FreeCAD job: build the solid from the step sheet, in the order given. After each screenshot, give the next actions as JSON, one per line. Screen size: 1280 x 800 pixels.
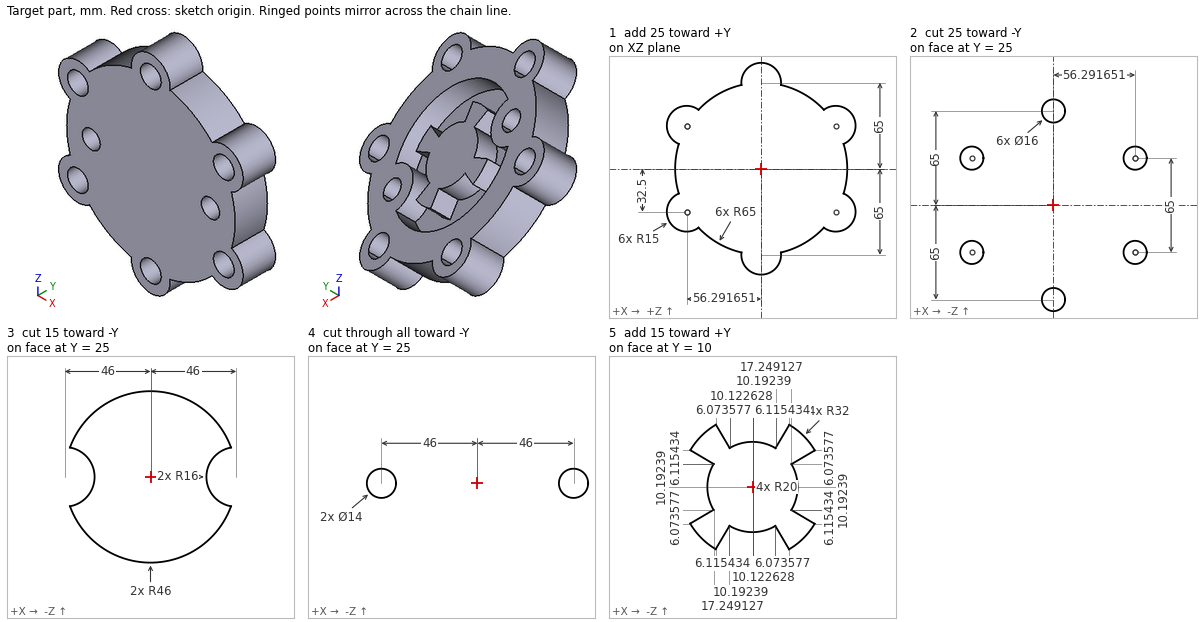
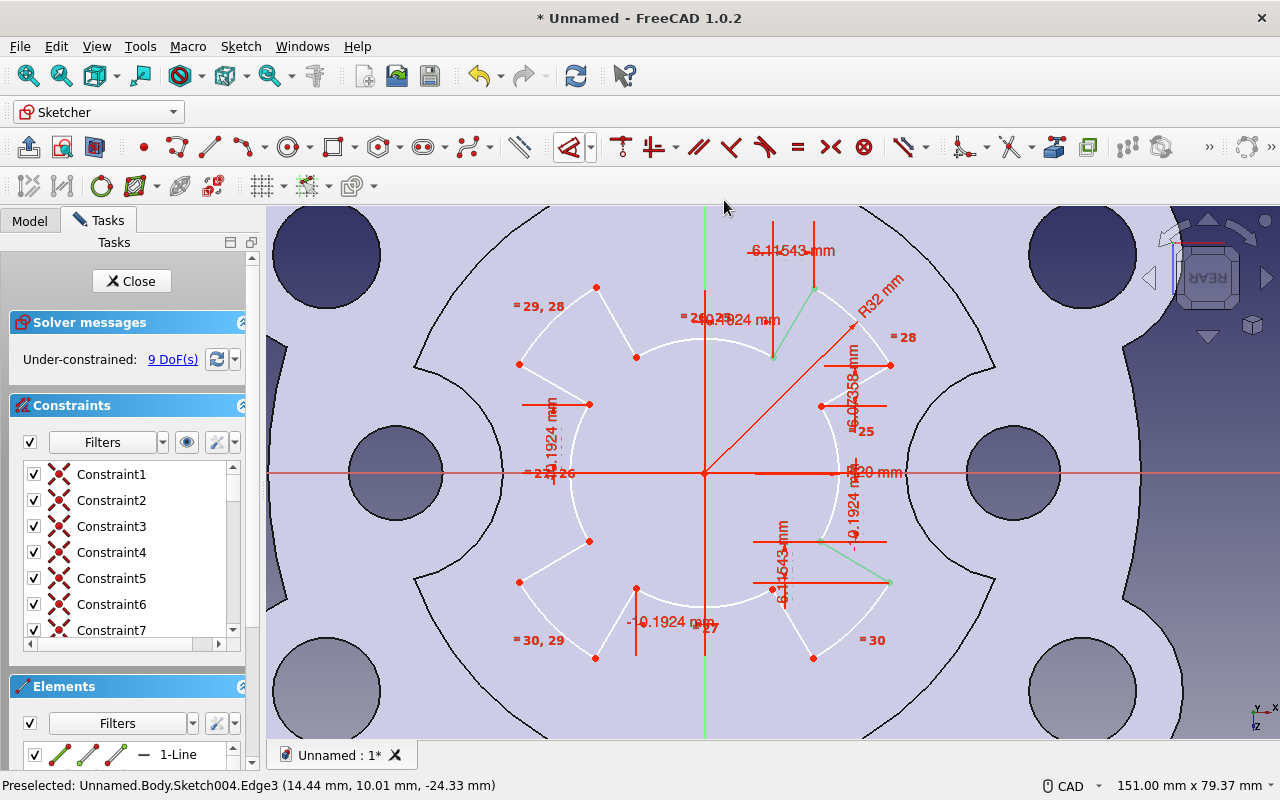
{"action": "left_click", "coordinate": [624, 337]}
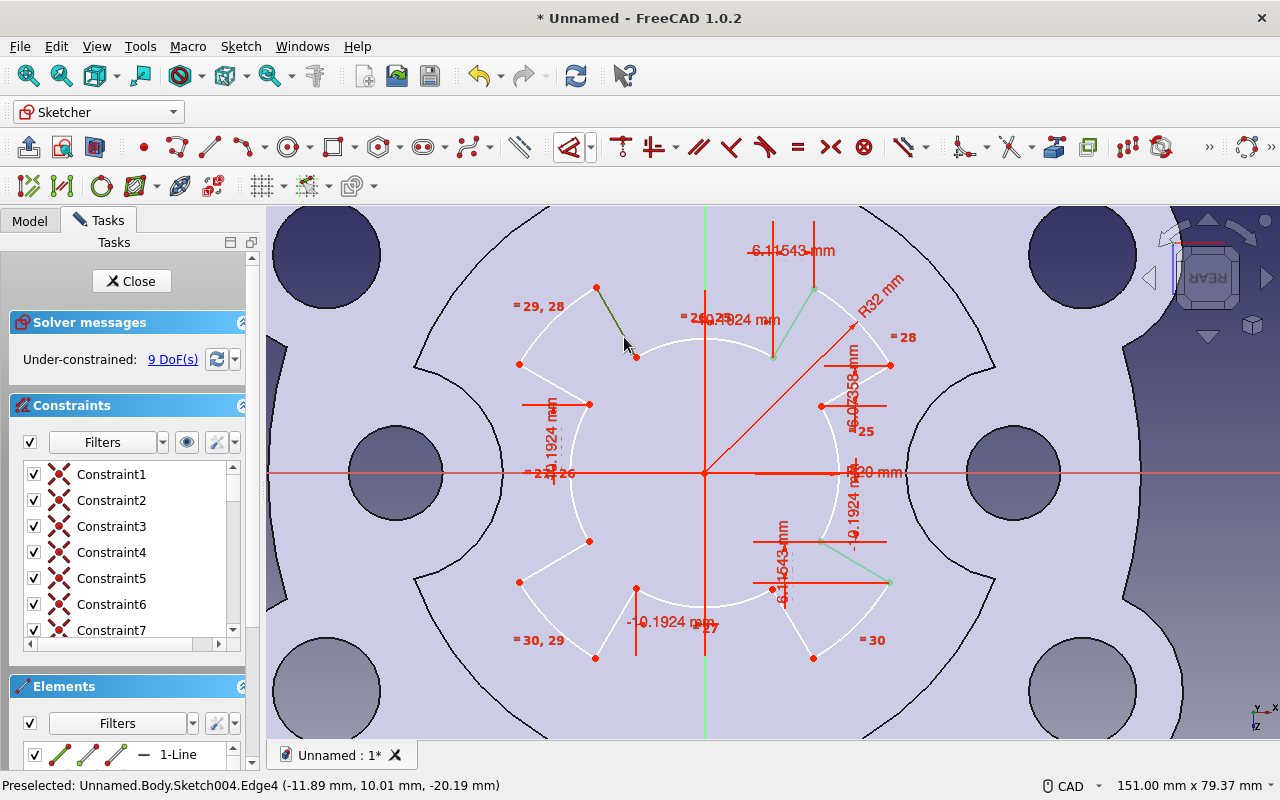
{"action": "left_click", "coordinate": [590, 148]}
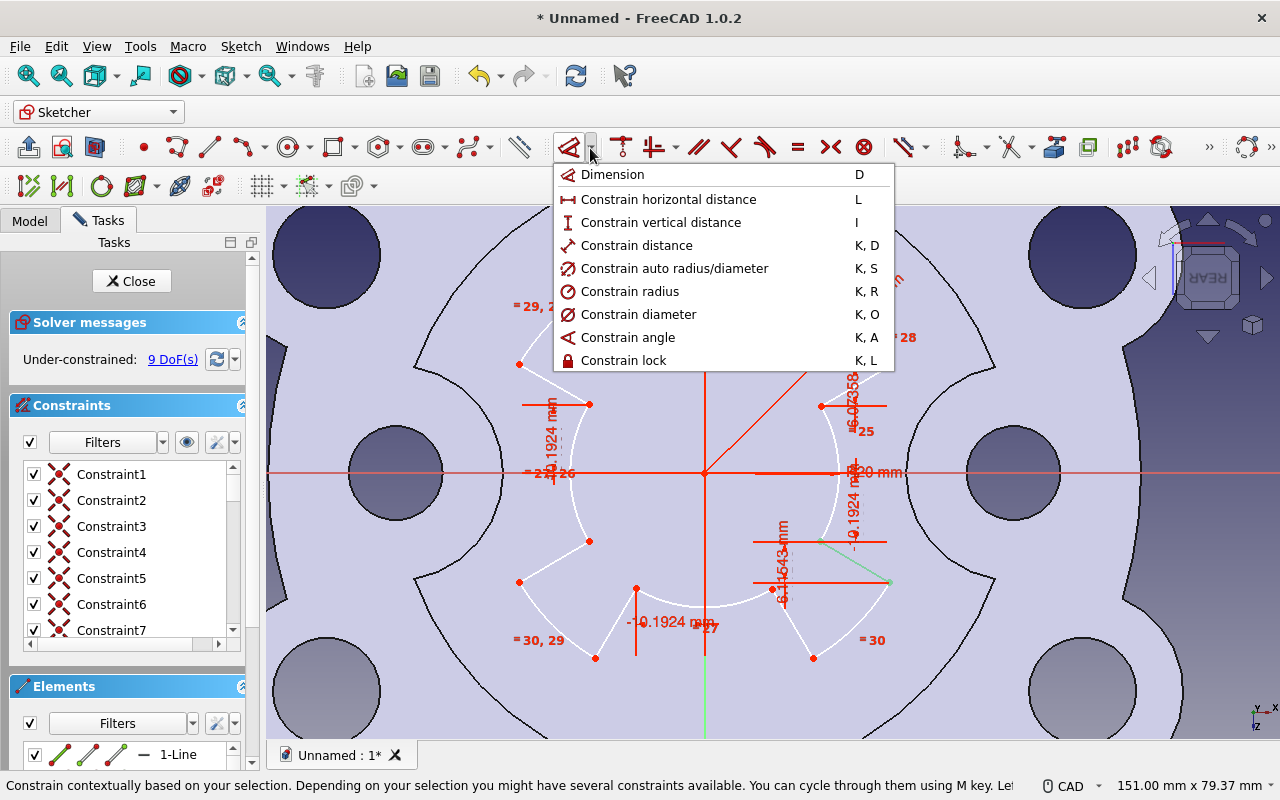
{"action": "left_click", "coordinate": [724, 200]}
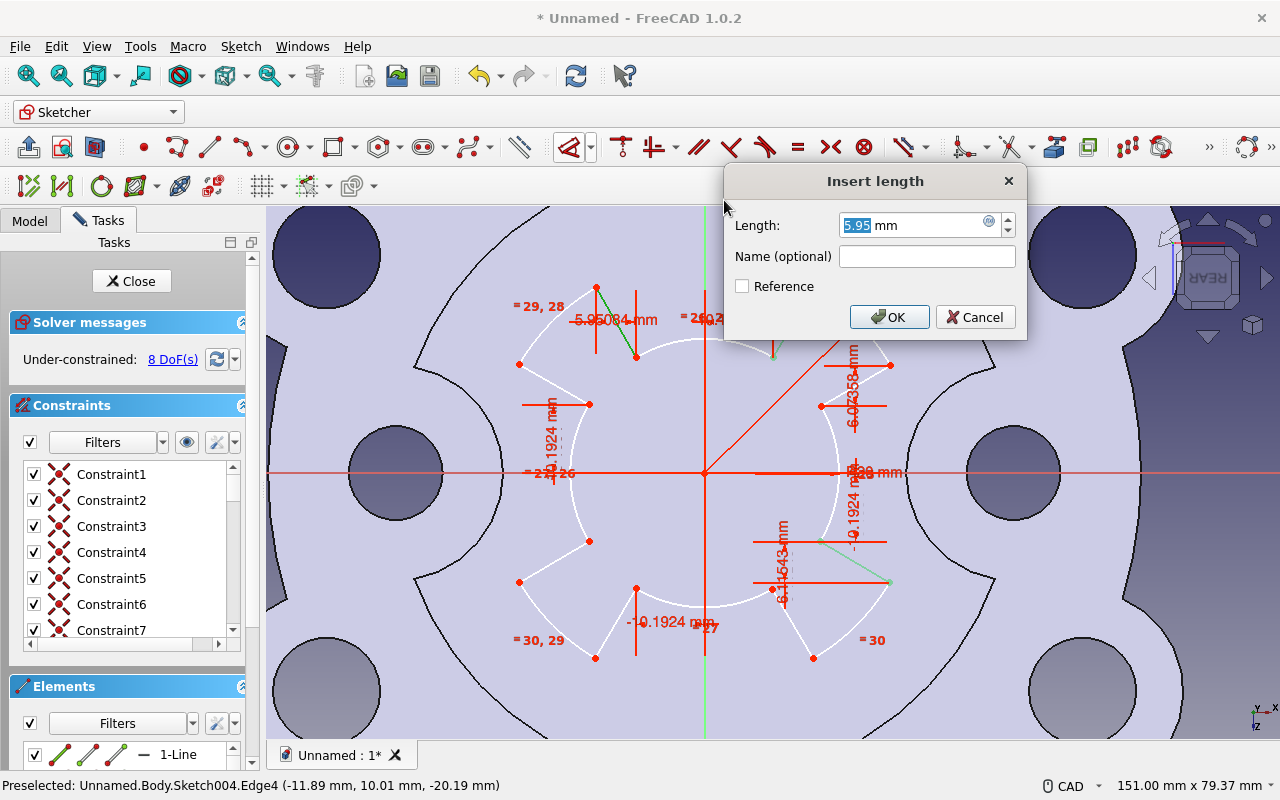
{"action": "type", "text": "6.073577"}
{"action": "key", "text": "Return"}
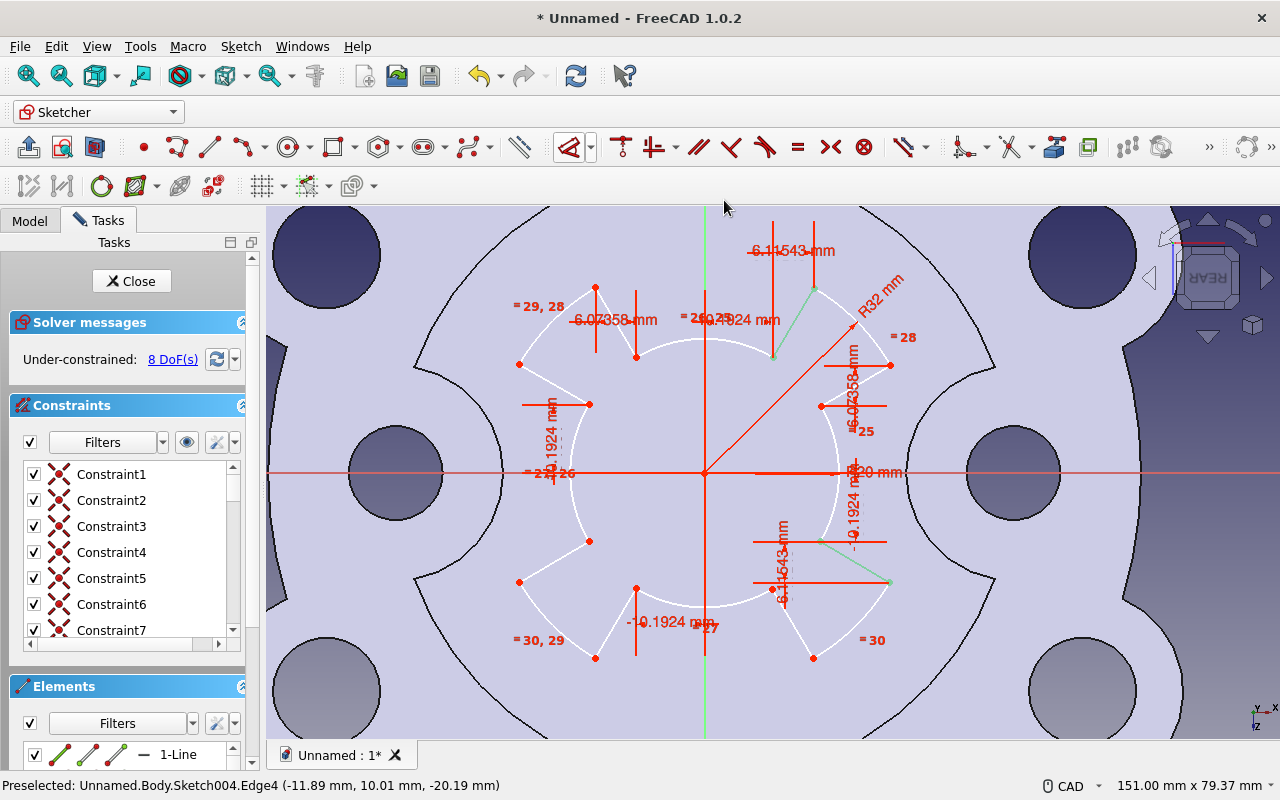
{"action": "left_click", "coordinate": [540, 377]}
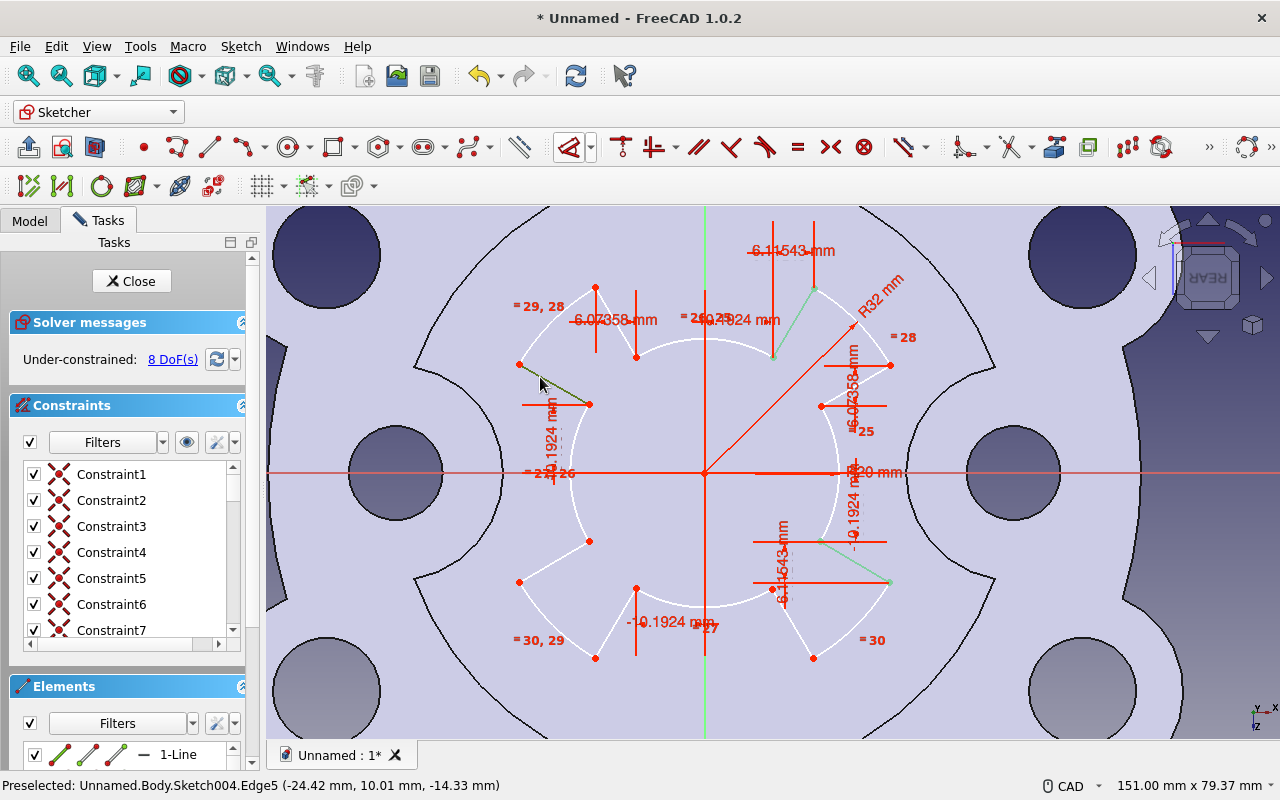
{"action": "key", "text": "i"}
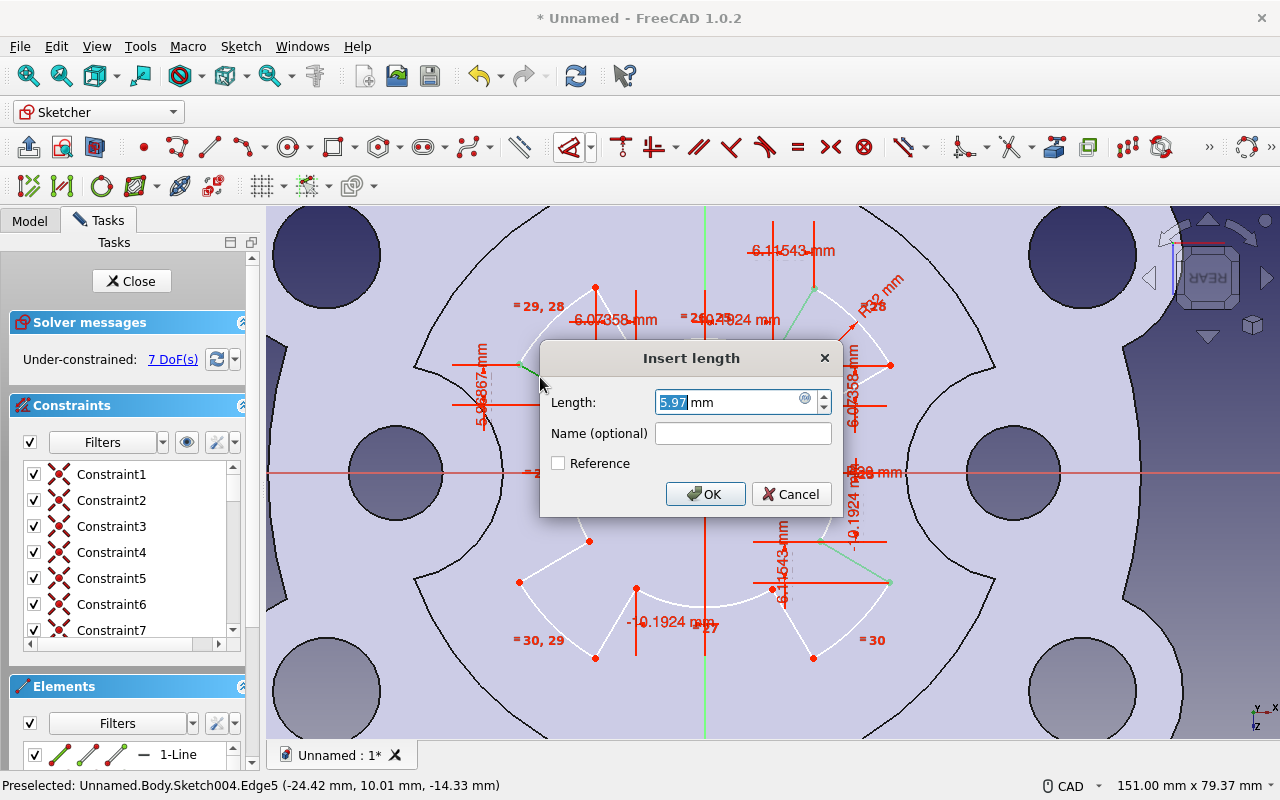
{"action": "type", "text": "6.115434"}
{"action": "key", "text": "Return"}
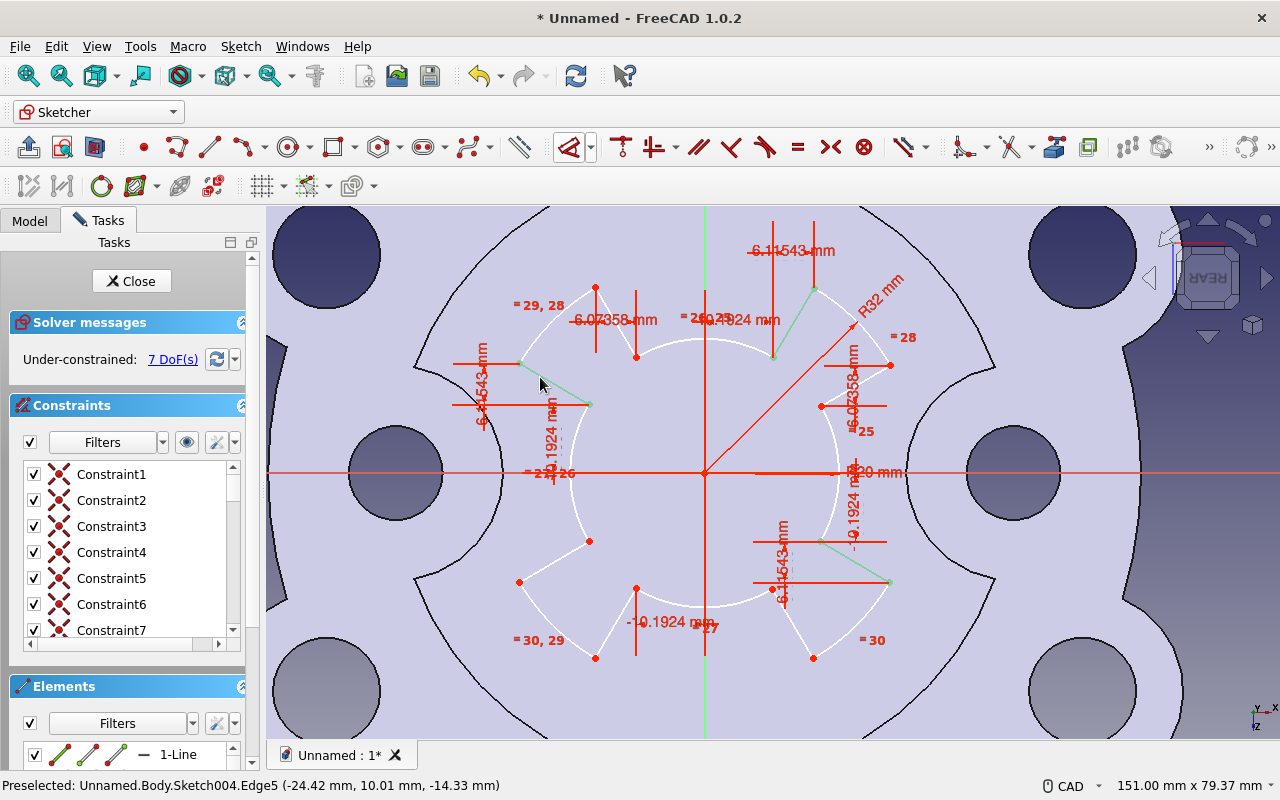
{"action": "left_click", "coordinate": [568, 554]}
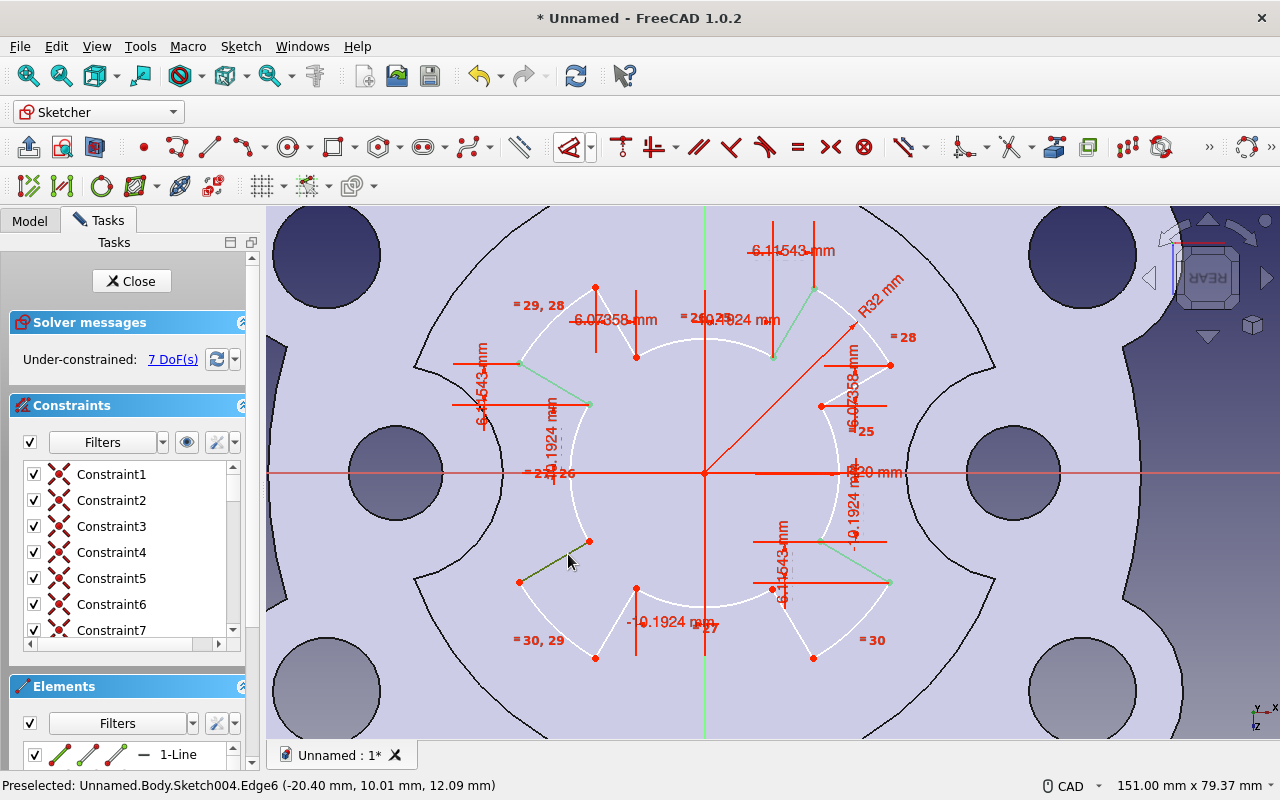
{"action": "left_click", "coordinate": [590, 148]}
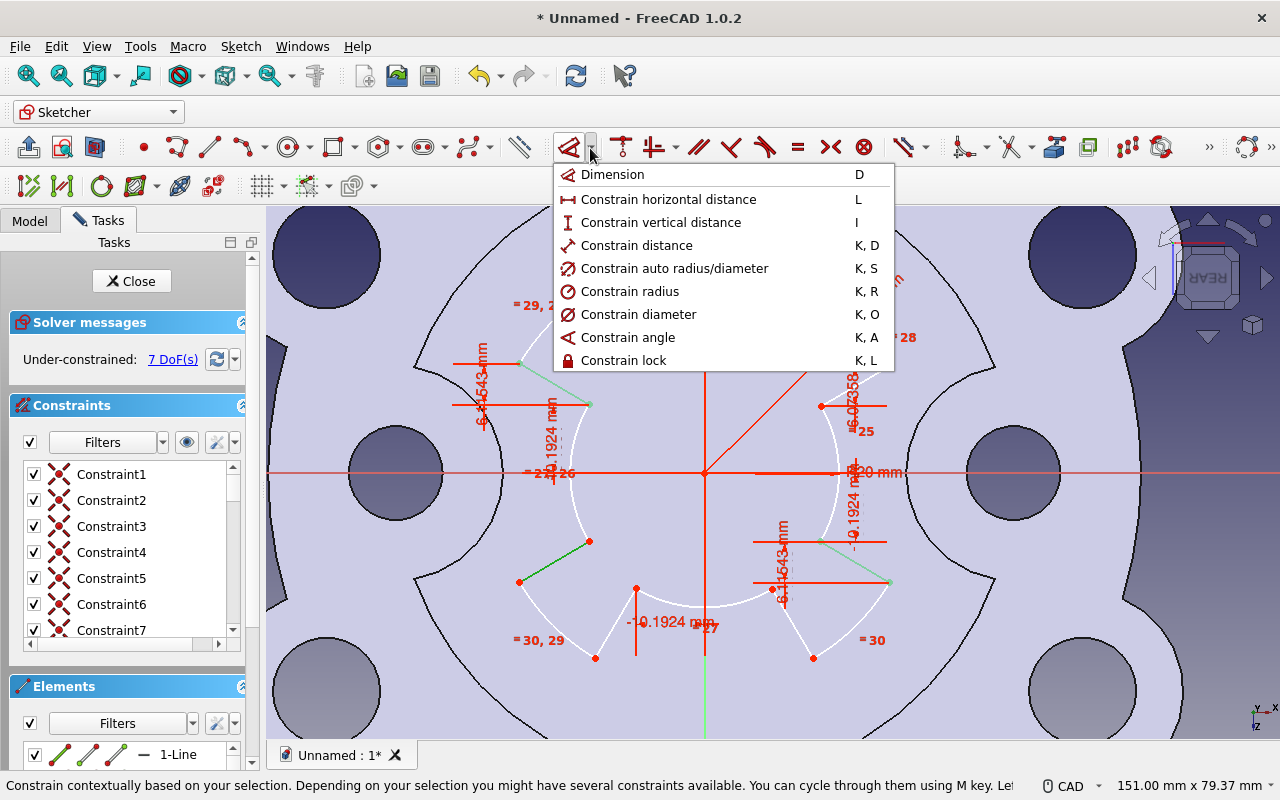
{"action": "left_click", "coordinate": [724, 222]}